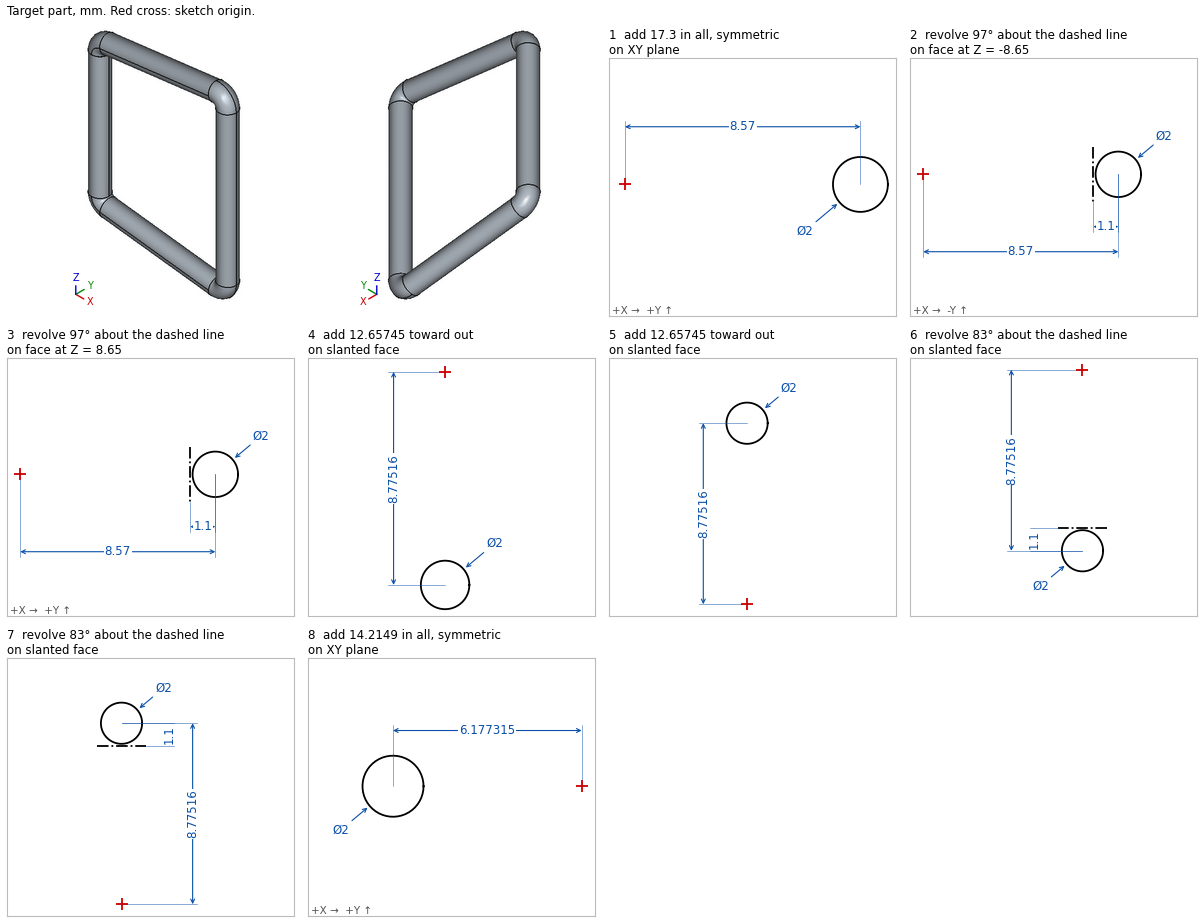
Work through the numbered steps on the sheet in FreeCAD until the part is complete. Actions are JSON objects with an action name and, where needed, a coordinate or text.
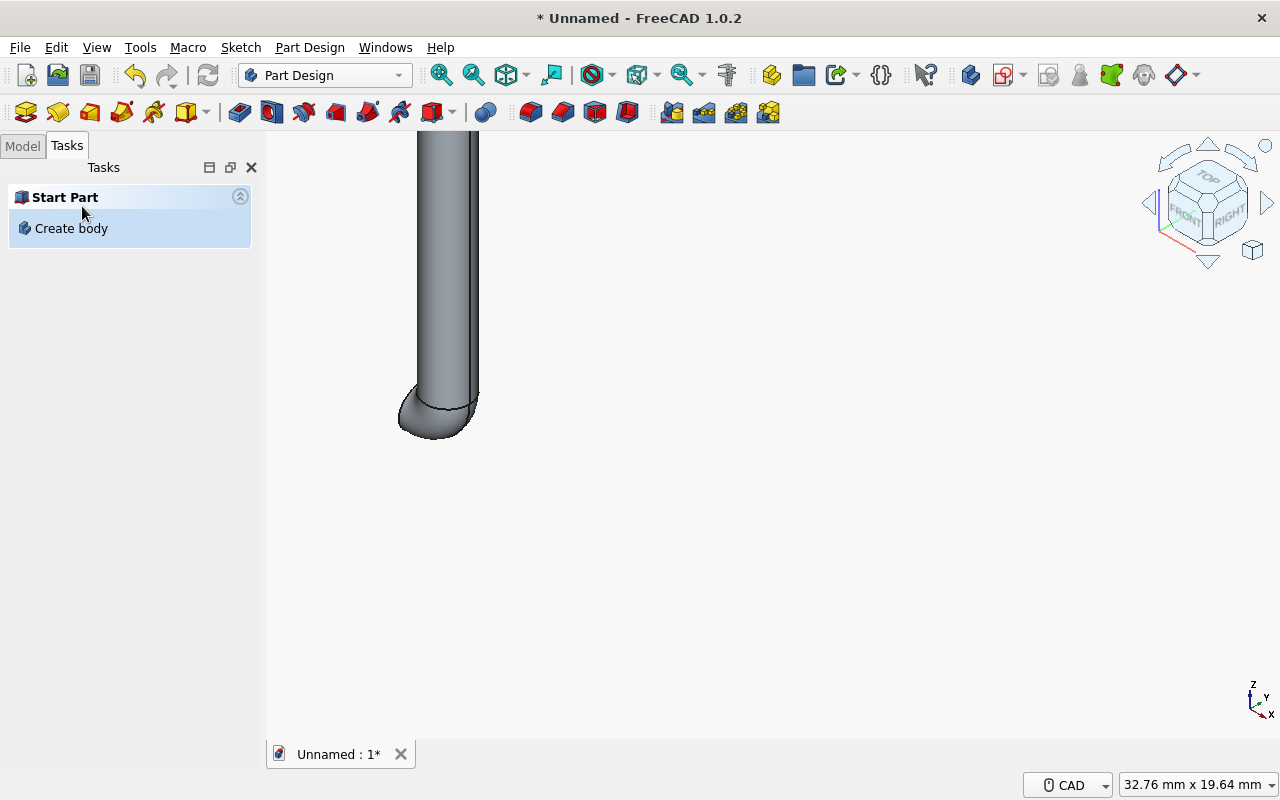
{"action": "left_click", "coordinate": [442, 76]}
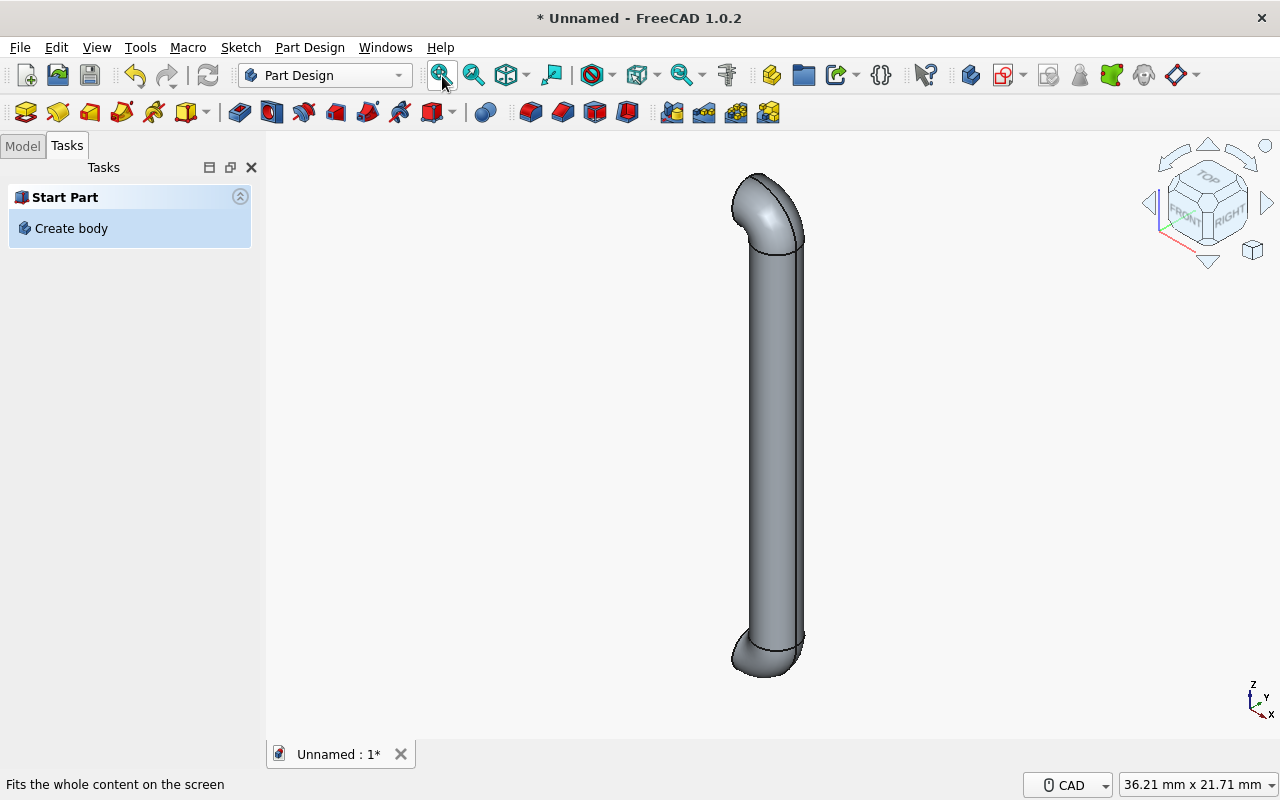
{"action": "key", "text": "6"}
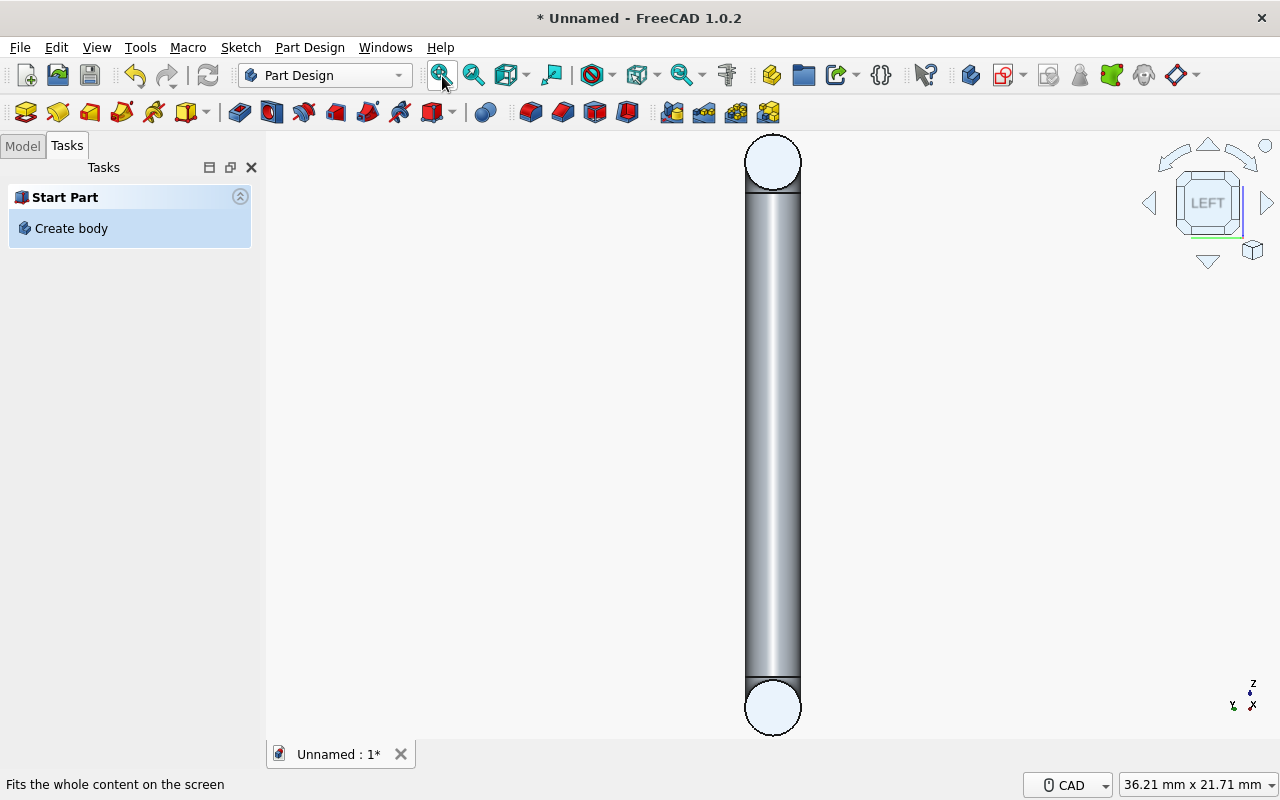
{"action": "left_click", "coordinate": [773, 707]}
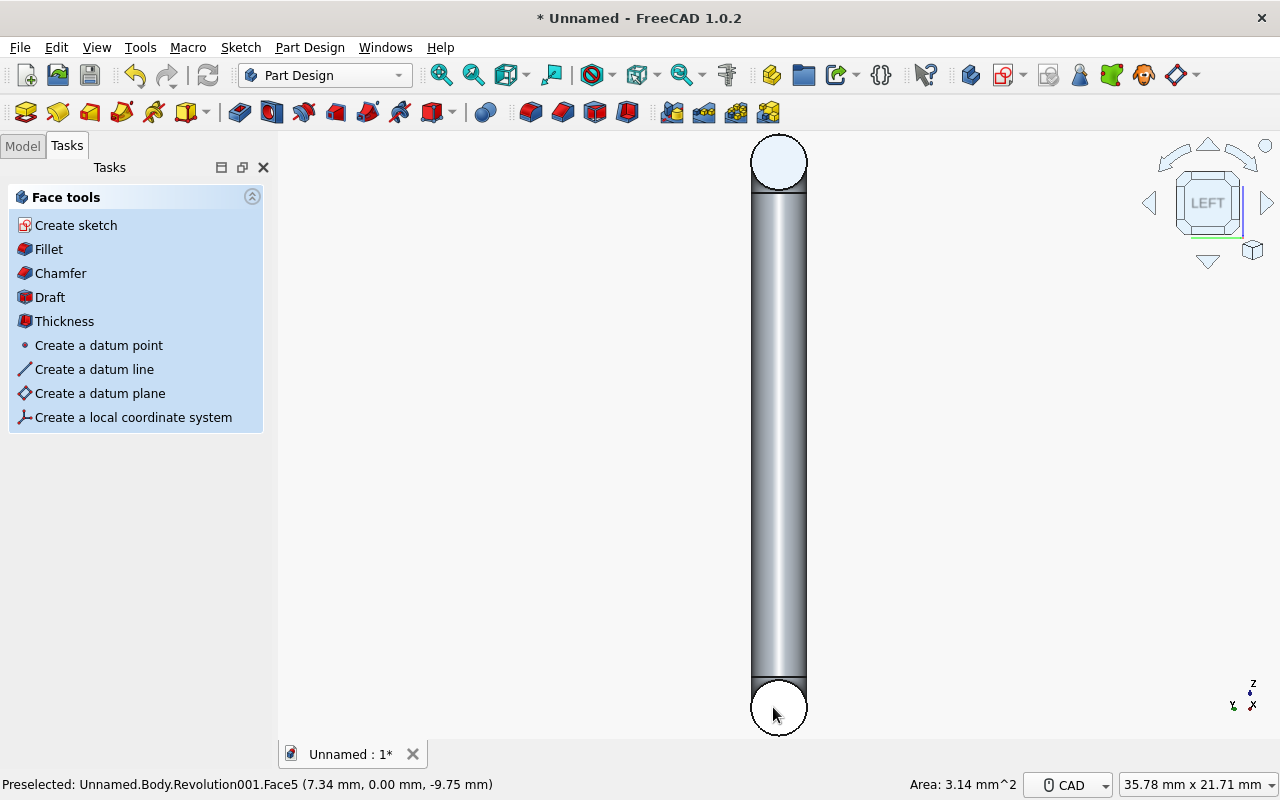
{"action": "left_click", "coordinate": [1004, 76]}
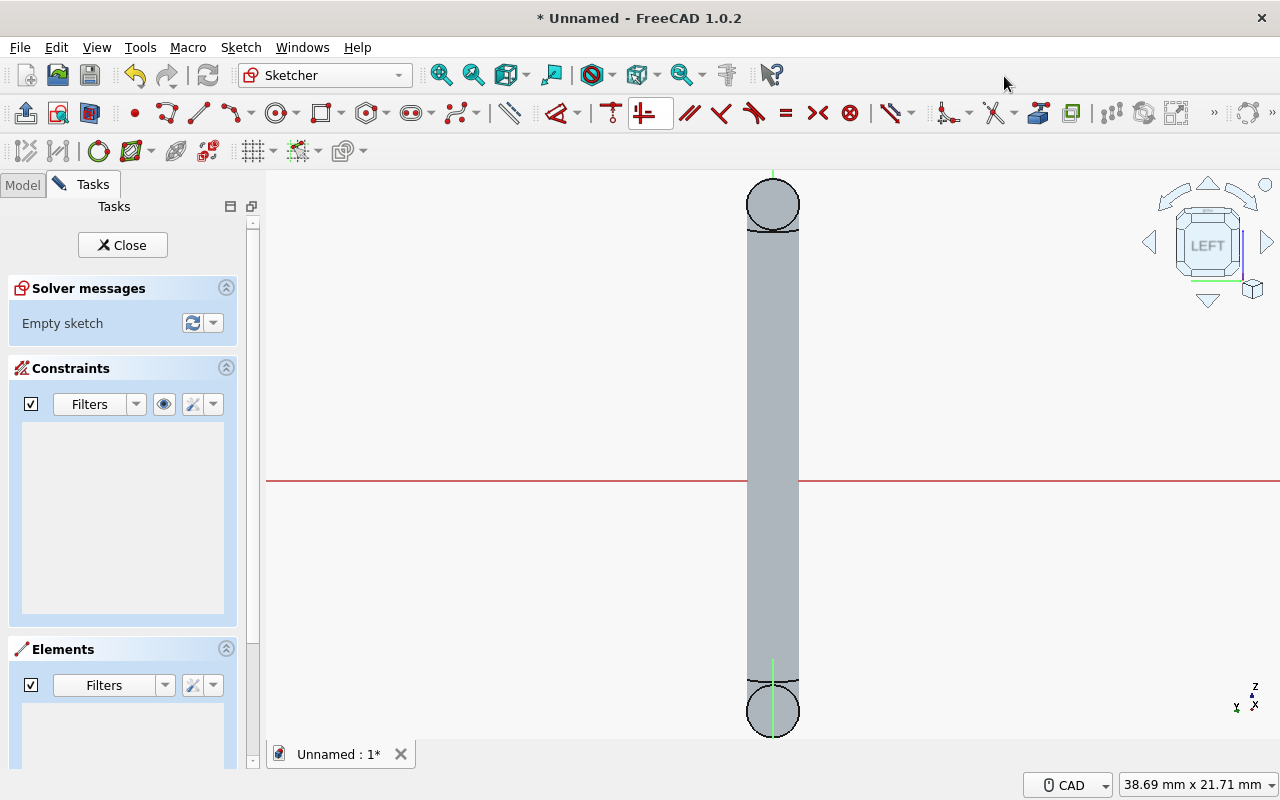
{"action": "scroll", "coordinate": [704, 454], "scroll_direction": "down", "scroll_amount": 5}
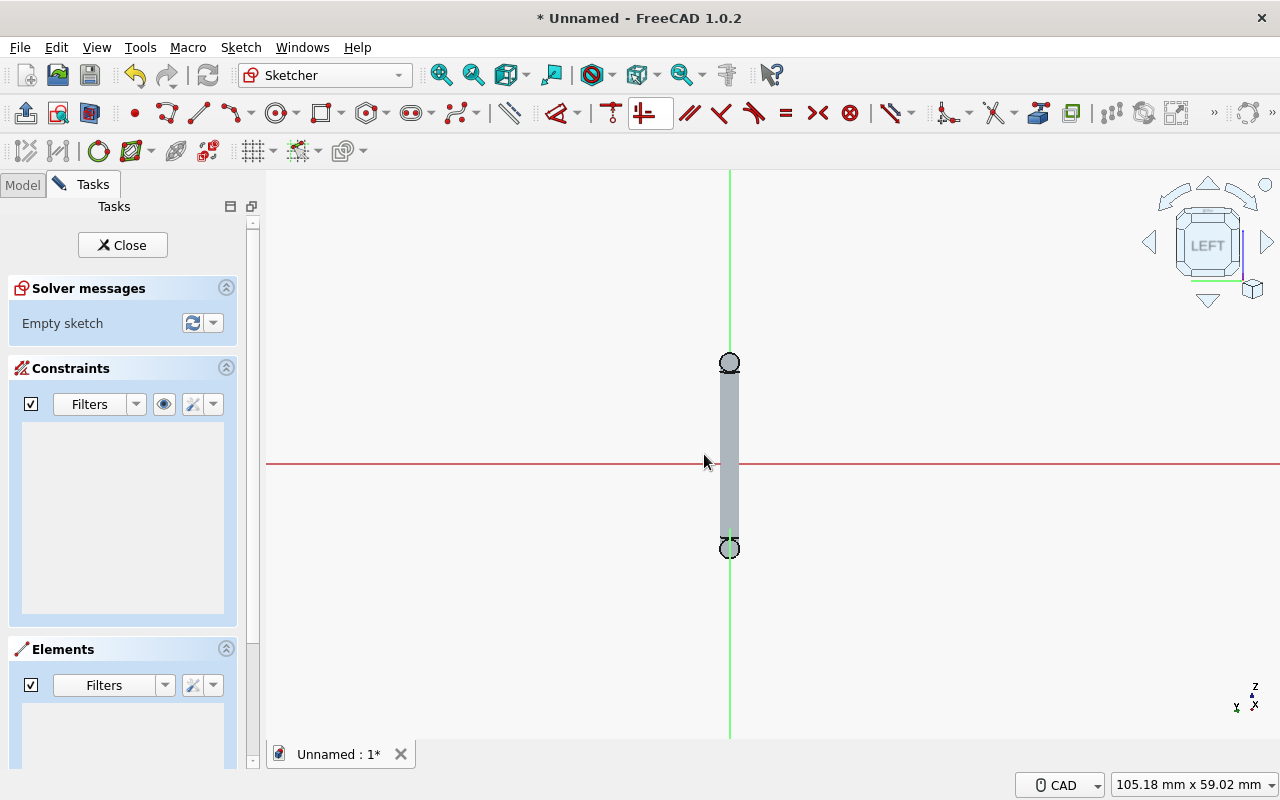
{"action": "scroll", "coordinate": [731, 554], "scroll_direction": "up", "scroll_amount": 15}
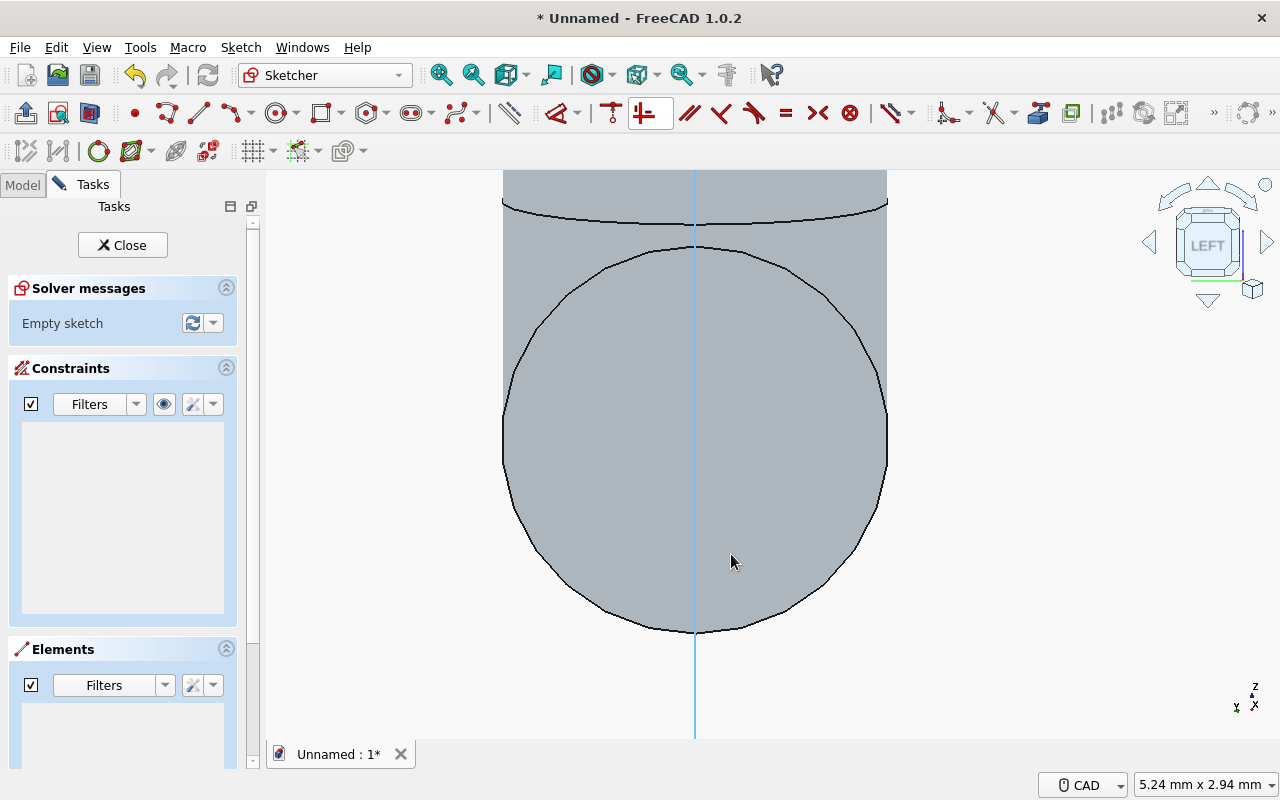
{"action": "left_click", "coordinate": [276, 114]}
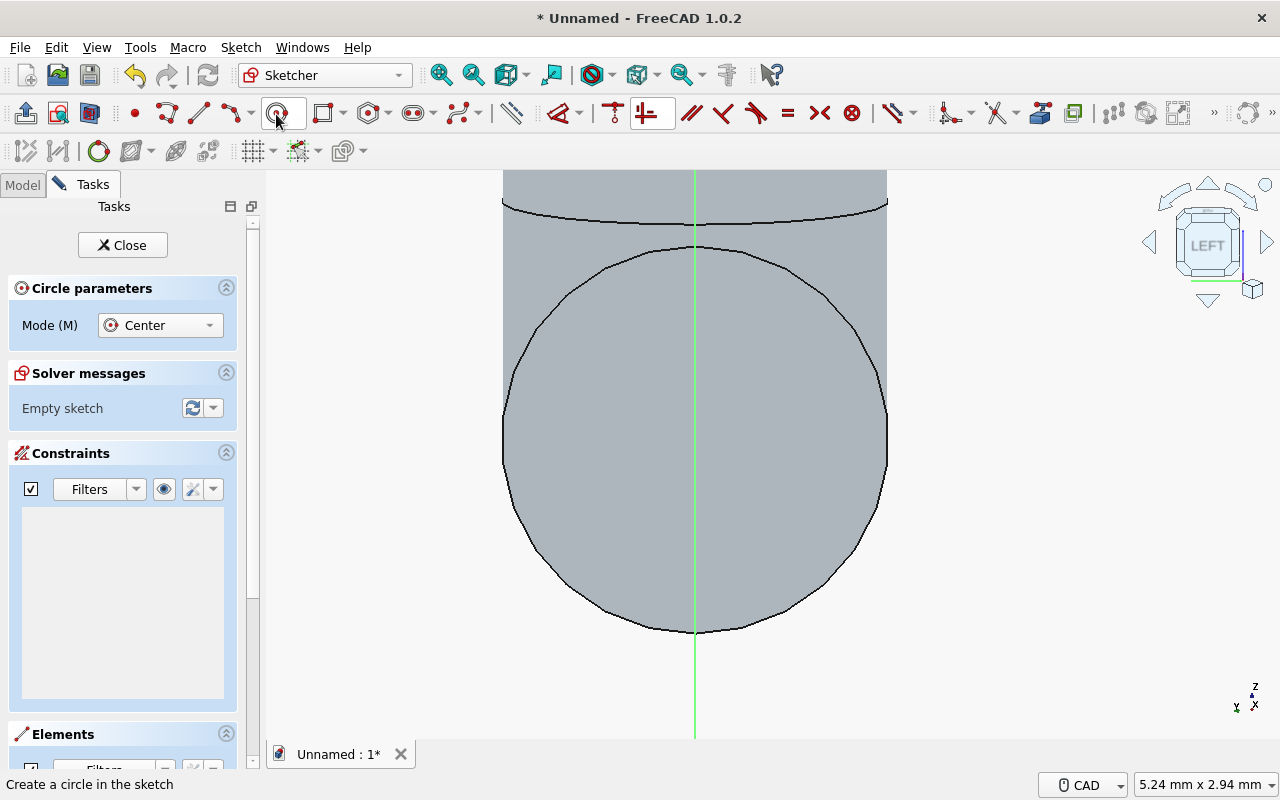
{"action": "left_click", "coordinate": [695, 440]}
{"action": "mouse_move", "coordinate": [832, 303]}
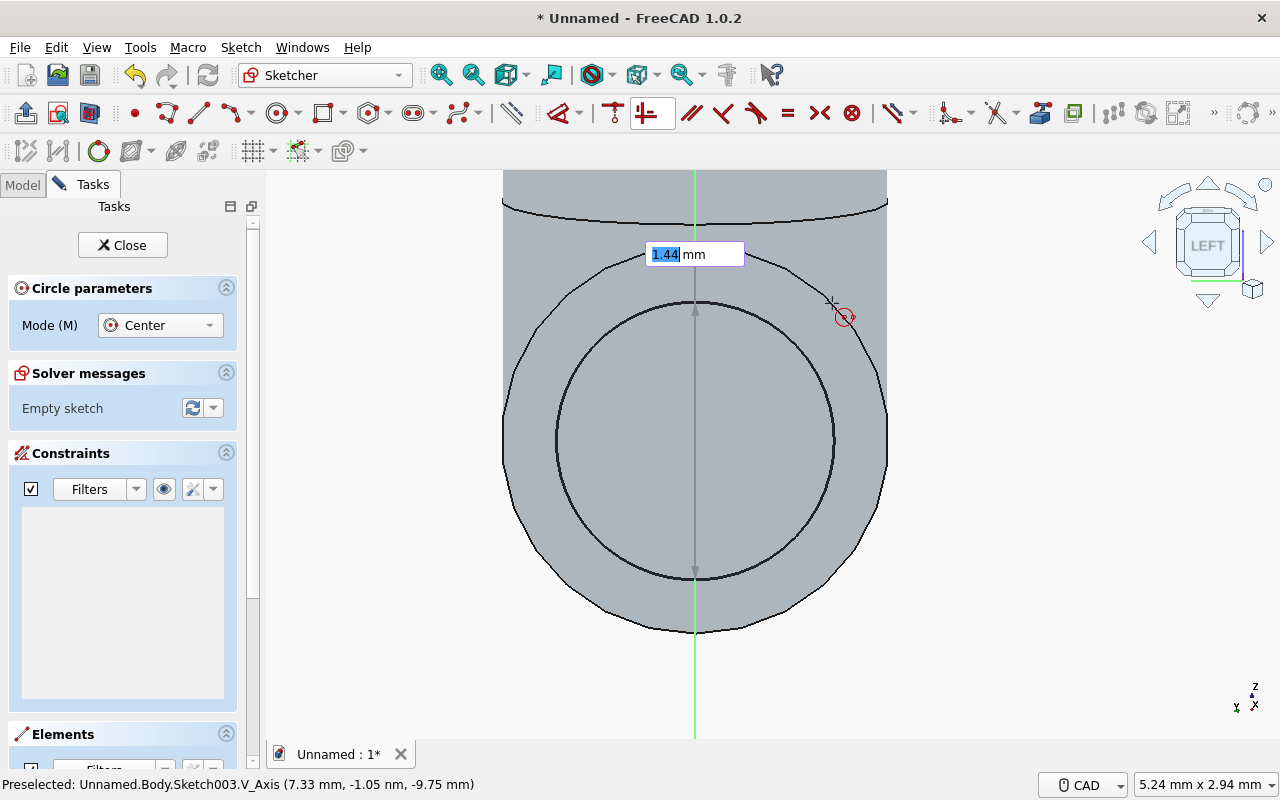
{"action": "type", "text": "2"}
{"action": "key", "text": "Return"}
{"action": "key", "text": "Escape"}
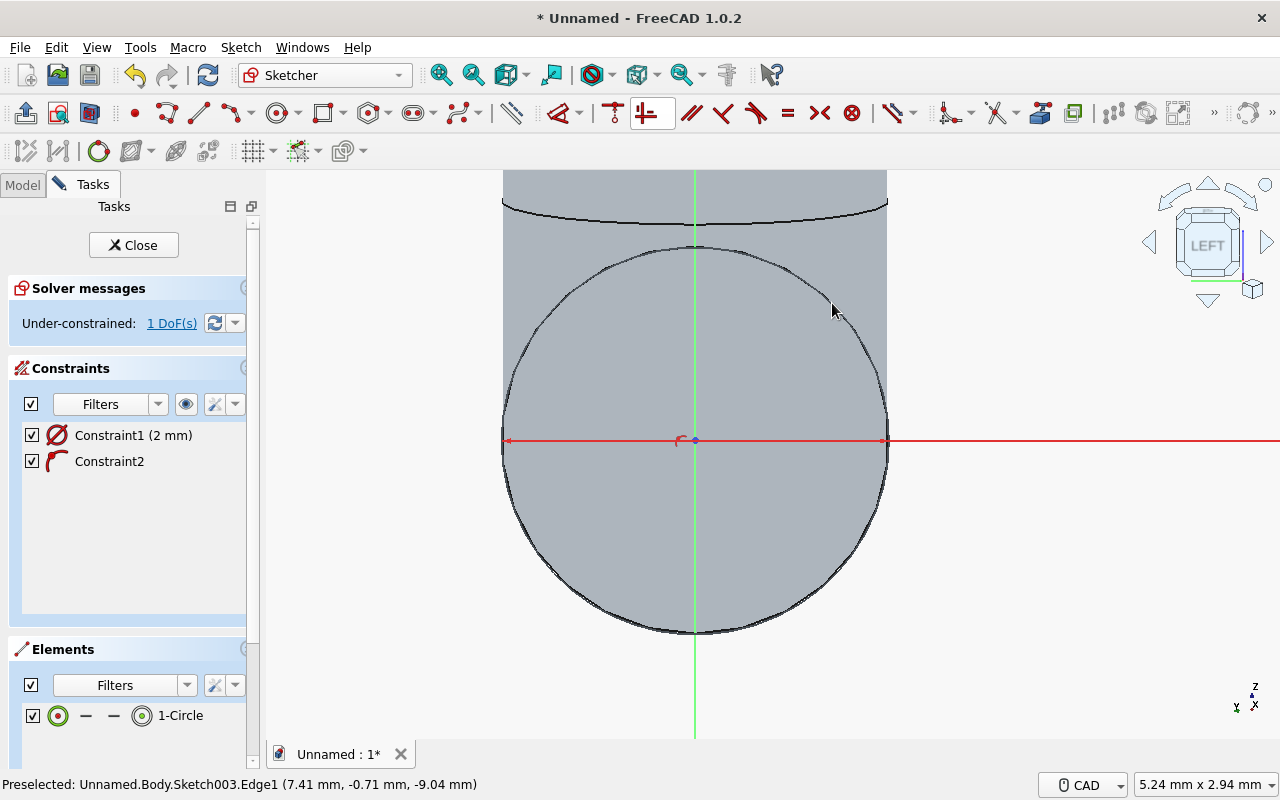
{"action": "left_click", "coordinate": [558, 114]}